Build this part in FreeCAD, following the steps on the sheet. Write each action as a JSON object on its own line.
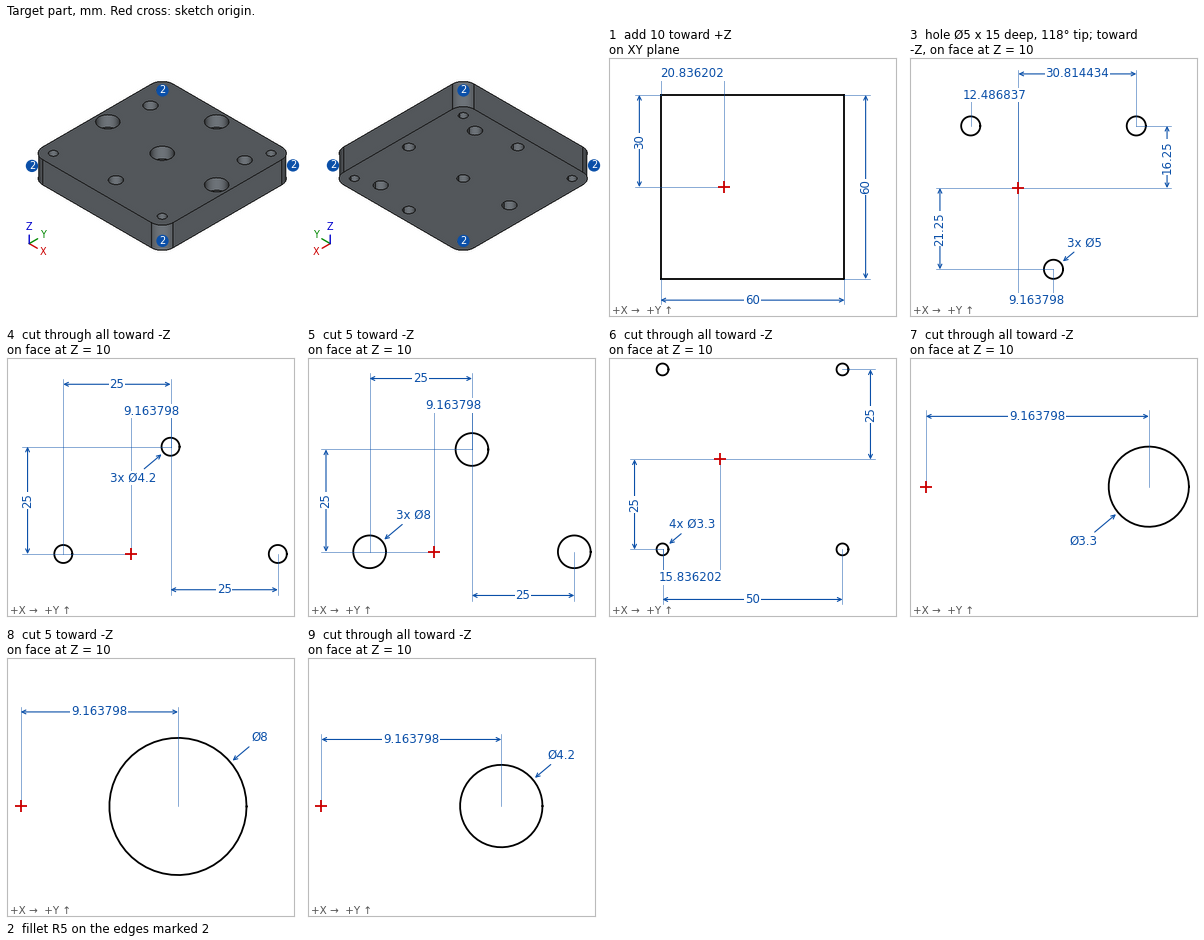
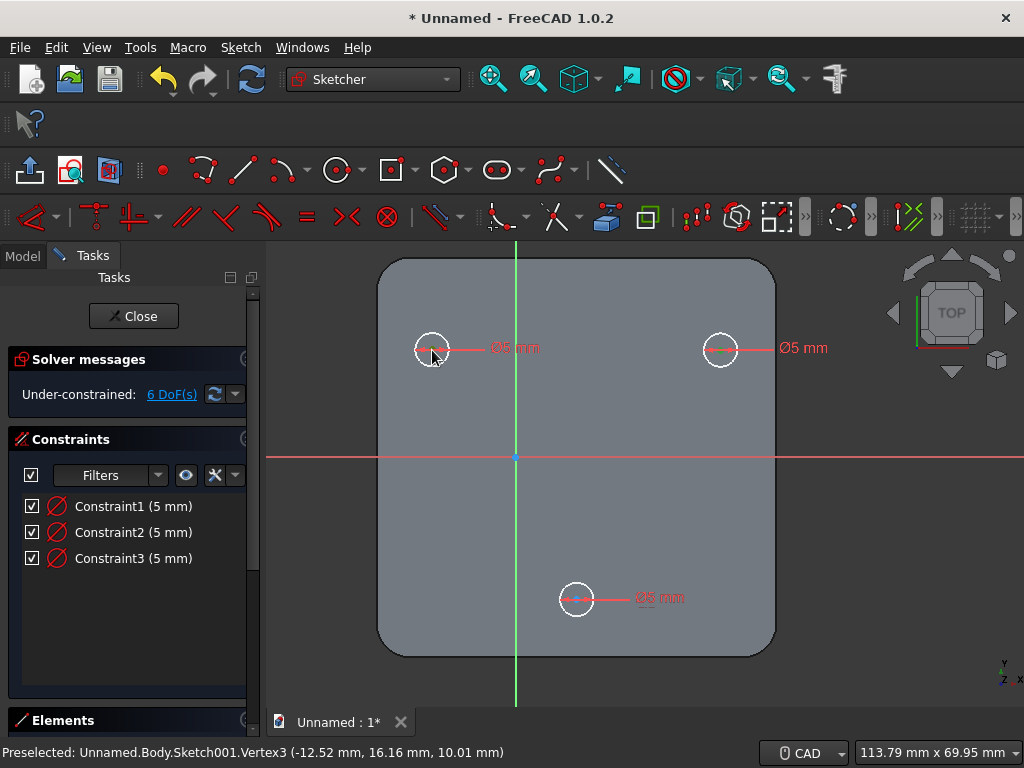
{"action": "key", "text": "h"}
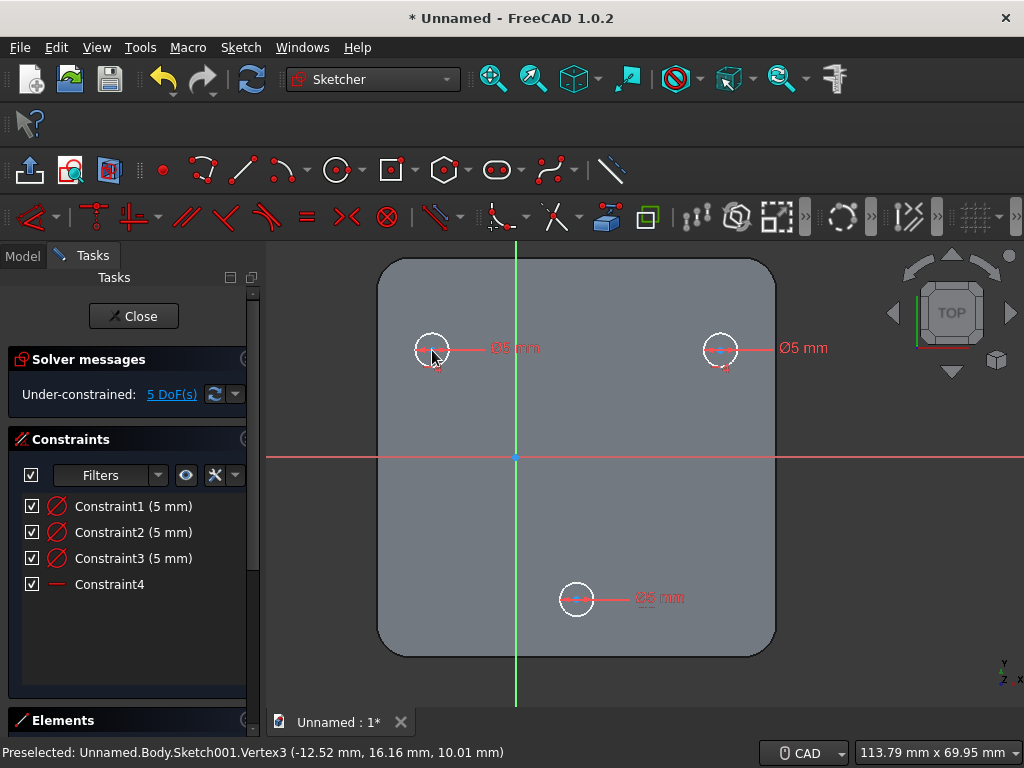
{"action": "left_click", "coordinate": [32, 218]}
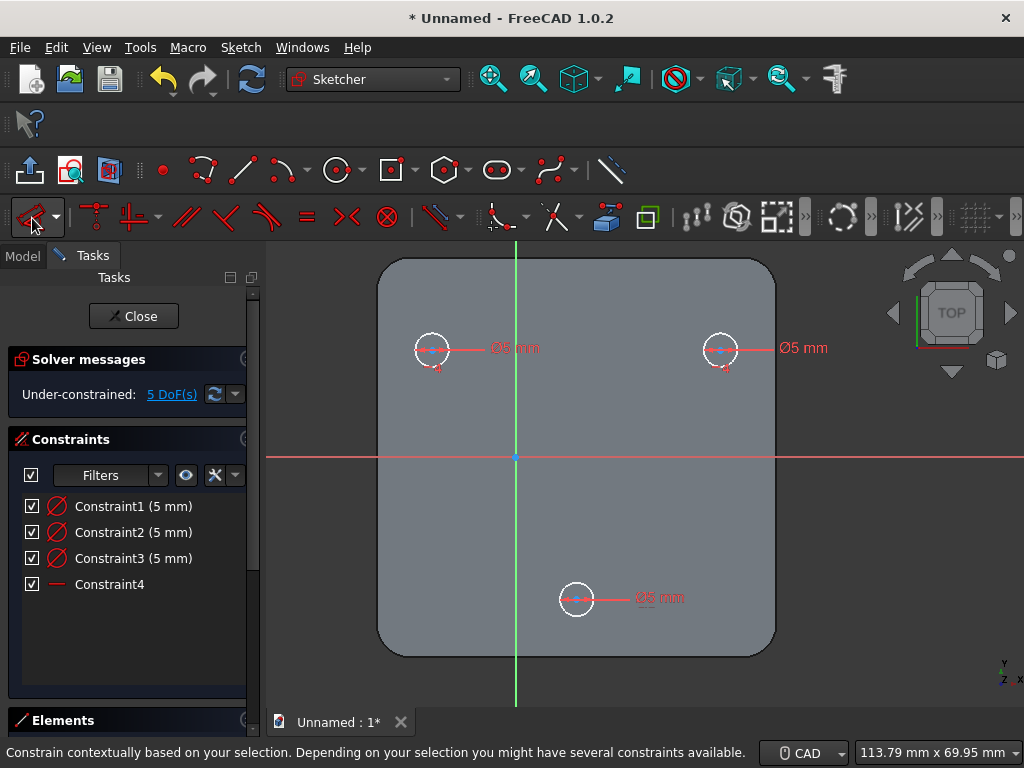
{"action": "left_click", "coordinate": [577, 599]}
{"action": "left_click", "coordinate": [482, 528]}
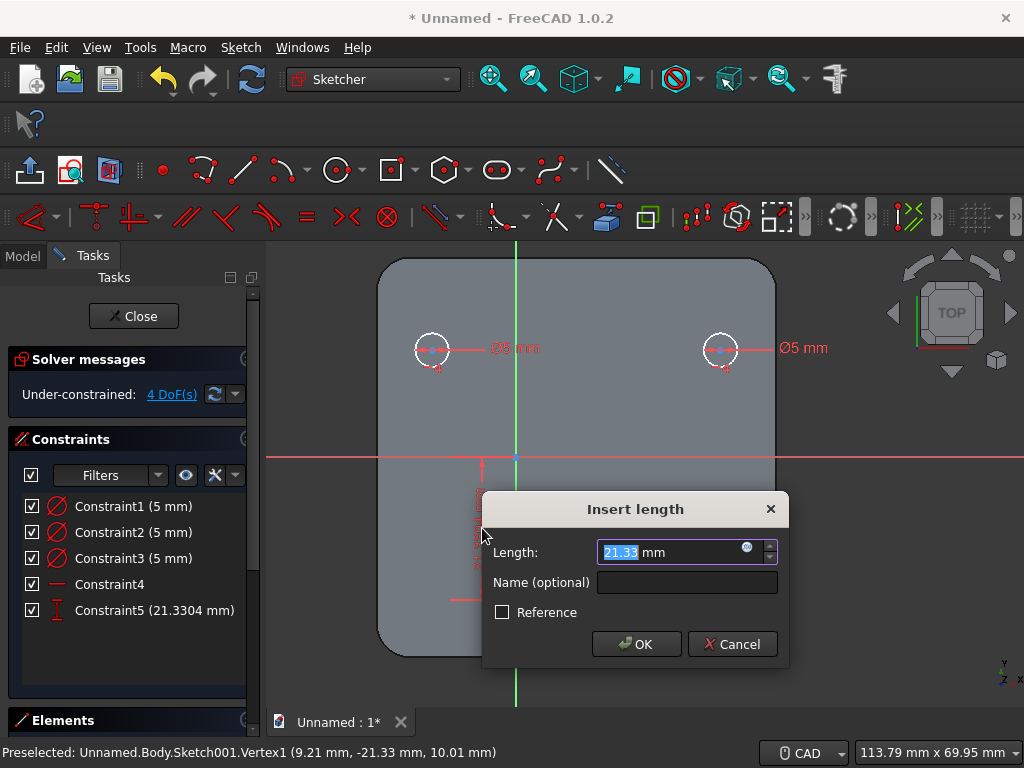
{"action": "type", "text": "21.25"}
{"action": "key", "text": "Return"}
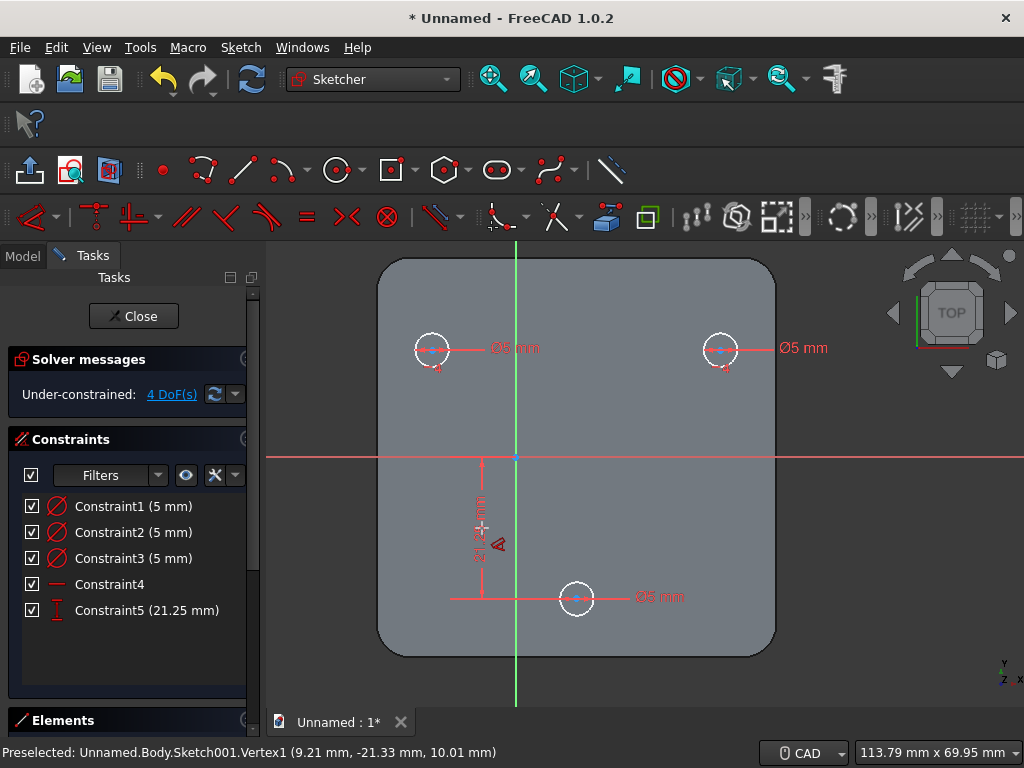
{"action": "left_click", "coordinate": [721, 350]}
{"action": "left_click", "coordinate": [755, 404]}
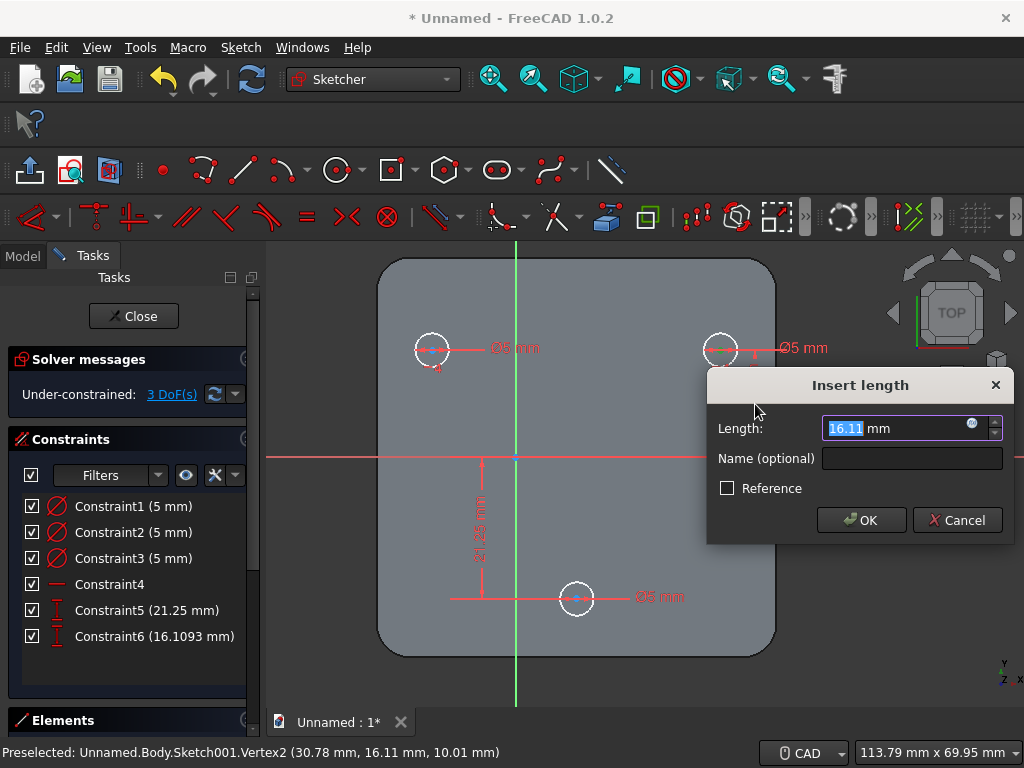
{"action": "type", "text": "16.25"}
{"action": "key", "text": "Return"}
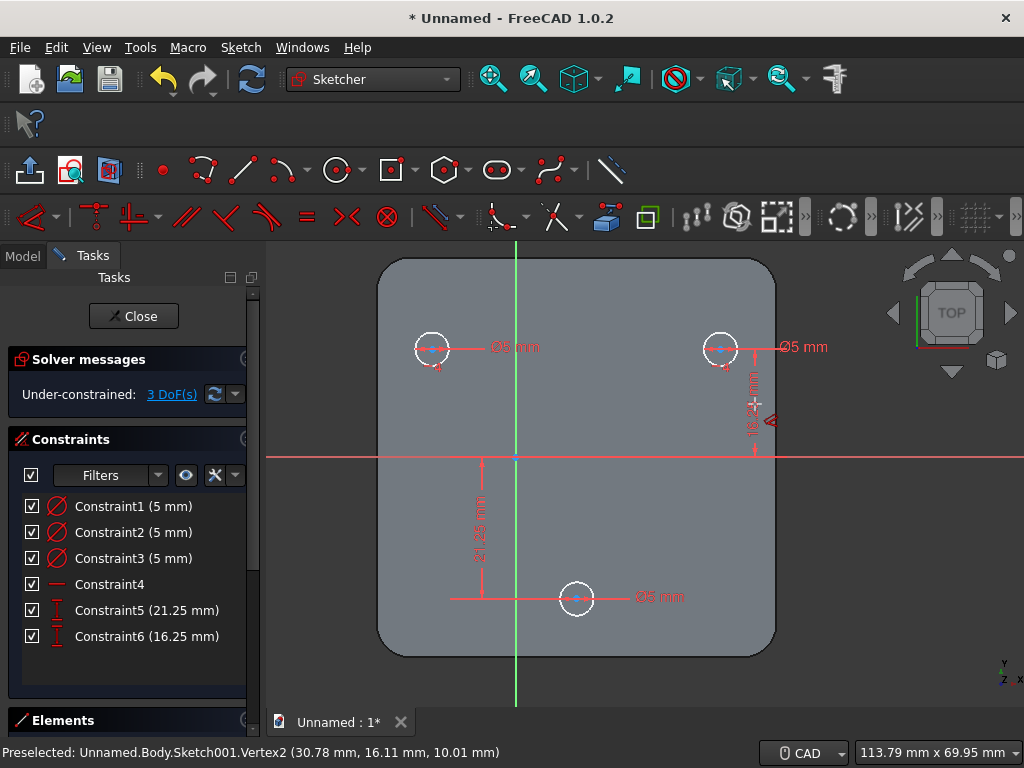
{"action": "left_click", "coordinate": [577, 599]}
{"action": "left_click", "coordinate": [546, 633]}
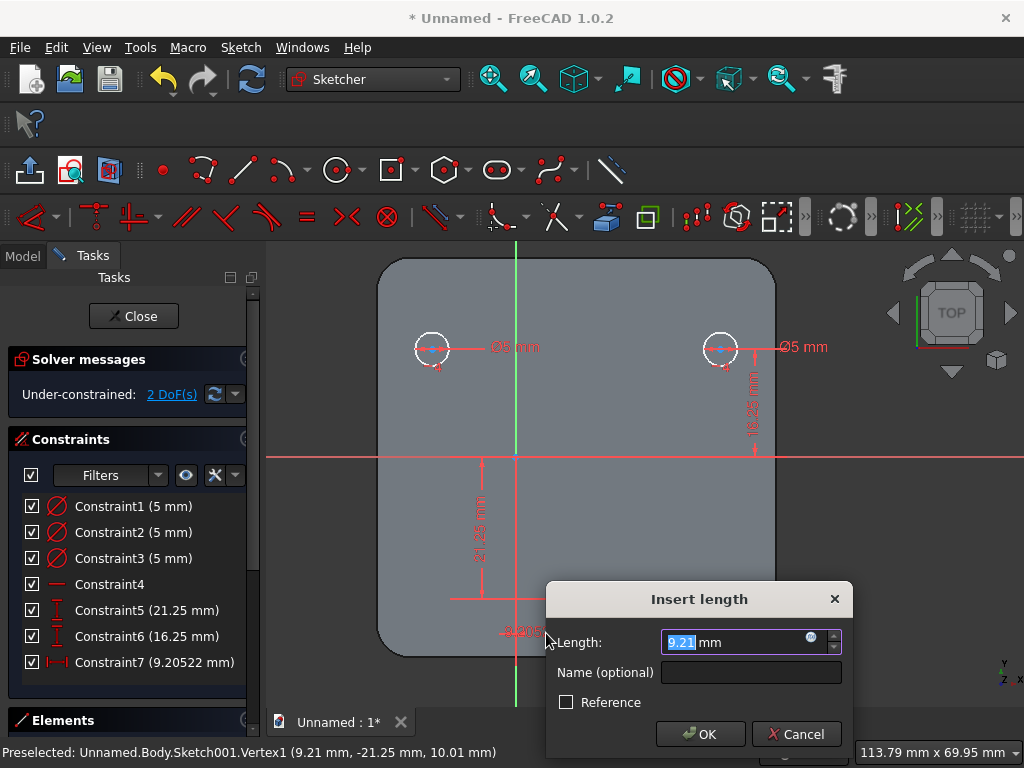
{"action": "type", "text": "9.163798"}
{"action": "key", "text": "Return"}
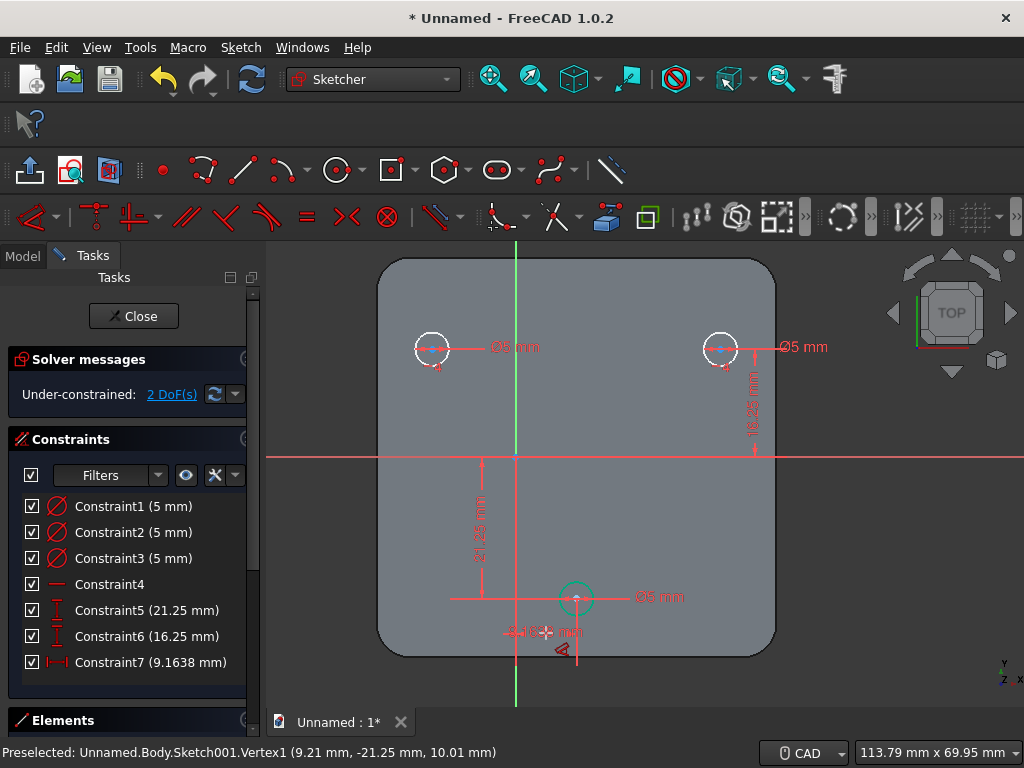
{"action": "left_click", "coordinate": [721, 349]}
{"action": "left_click", "coordinate": [618, 315]}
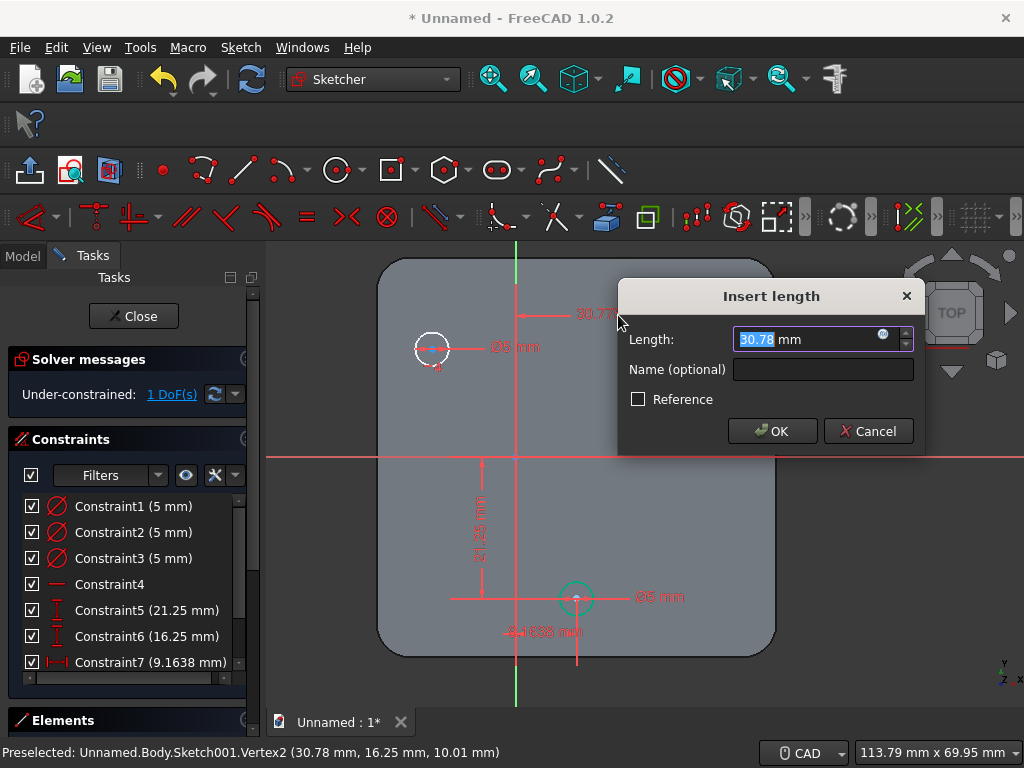
{"action": "type", "text": "30.814434"}
{"action": "key", "text": "Return"}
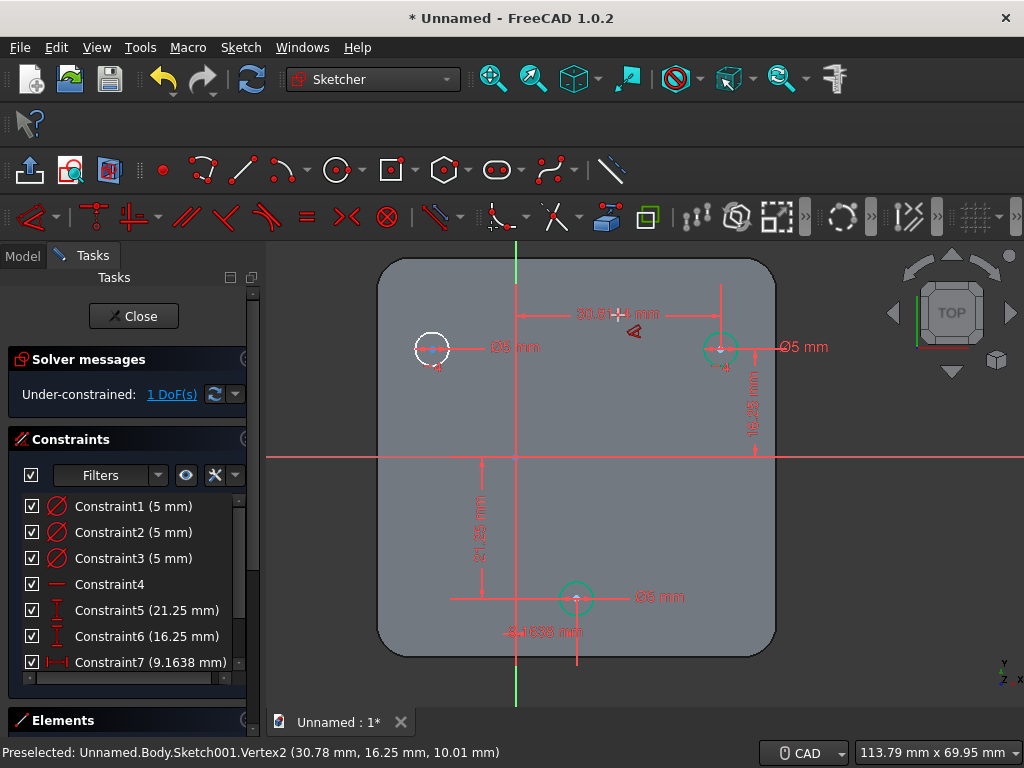
{"action": "left_click", "coordinate": [432, 349]}
{"action": "left_click", "coordinate": [474, 315]}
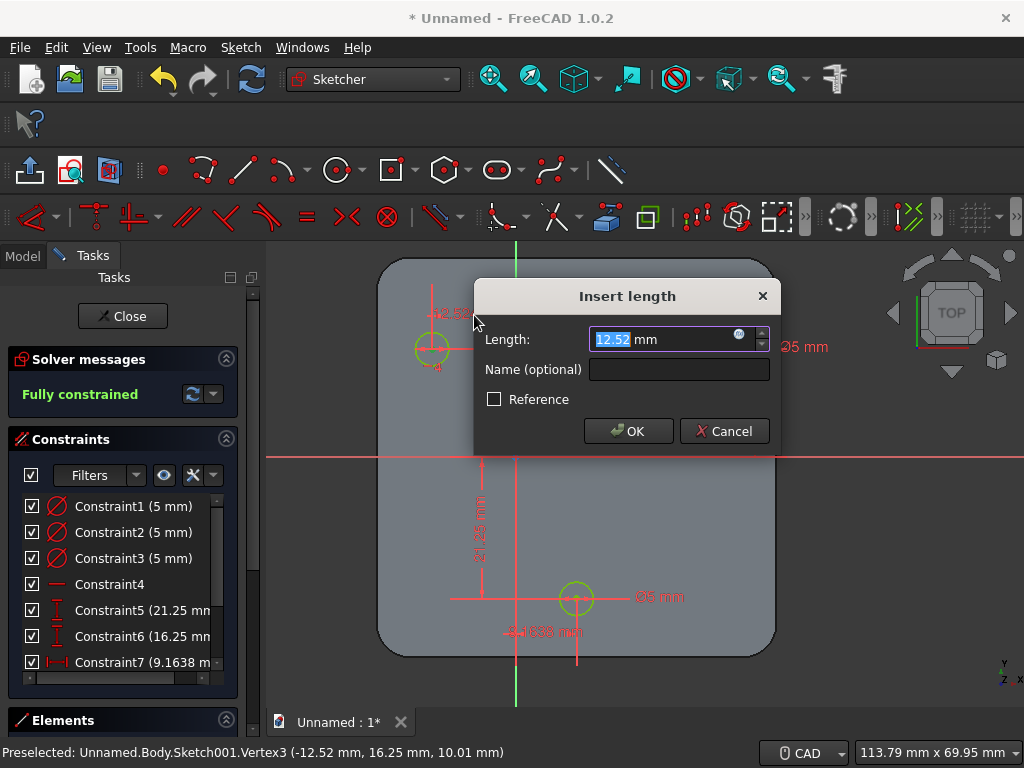
{"action": "type", "text": "12.486837"}
{"action": "key", "text": "Return"}
{"action": "key", "text": "Escape"}